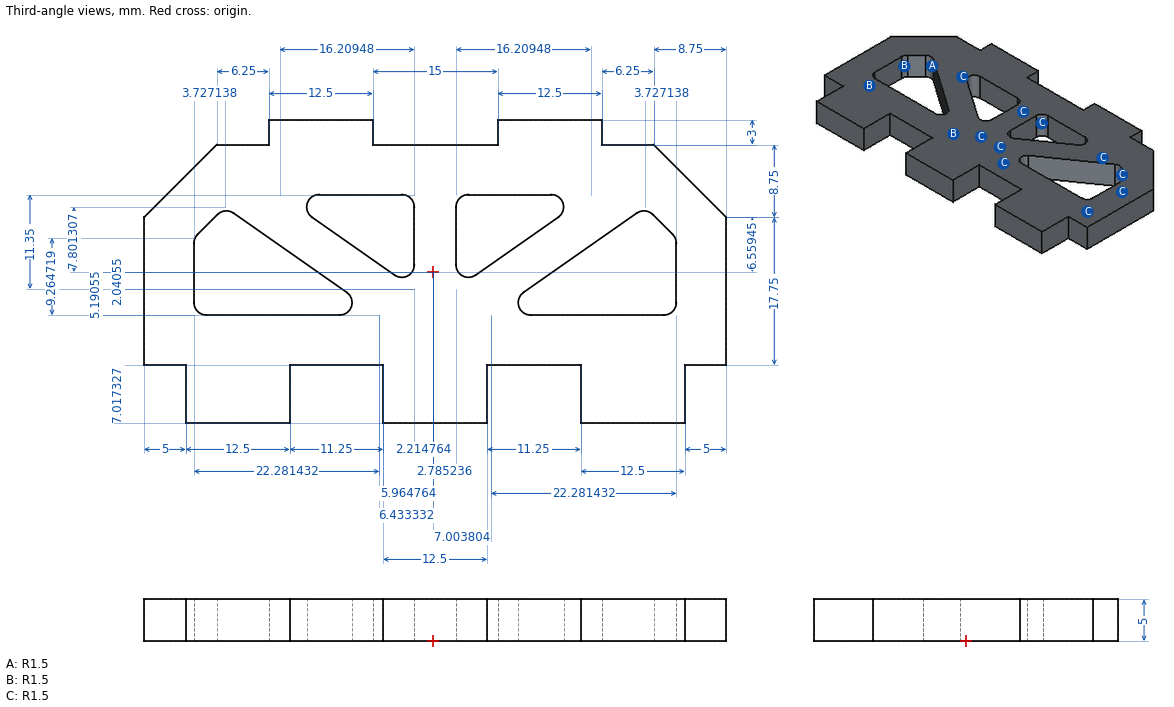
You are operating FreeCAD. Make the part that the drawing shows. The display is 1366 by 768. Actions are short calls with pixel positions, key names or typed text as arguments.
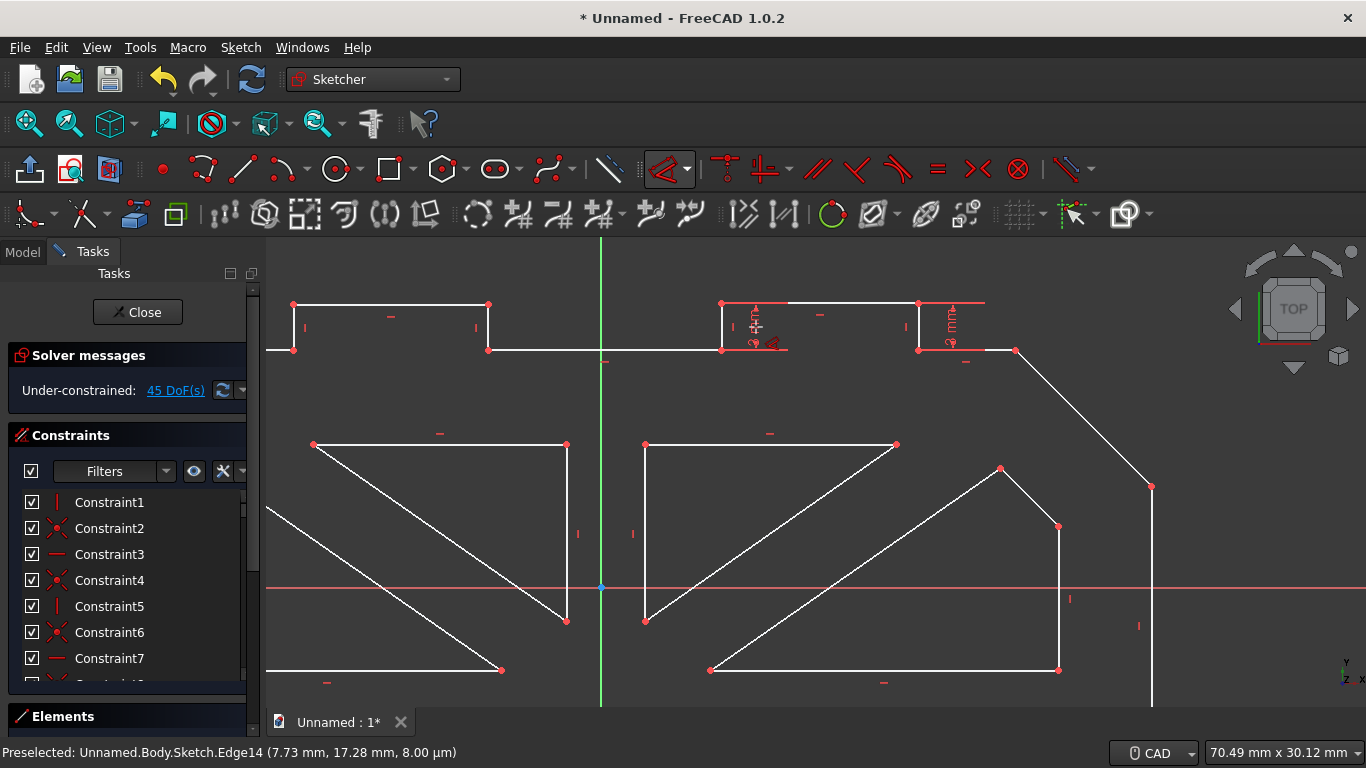
click(488, 336)
click(454, 327)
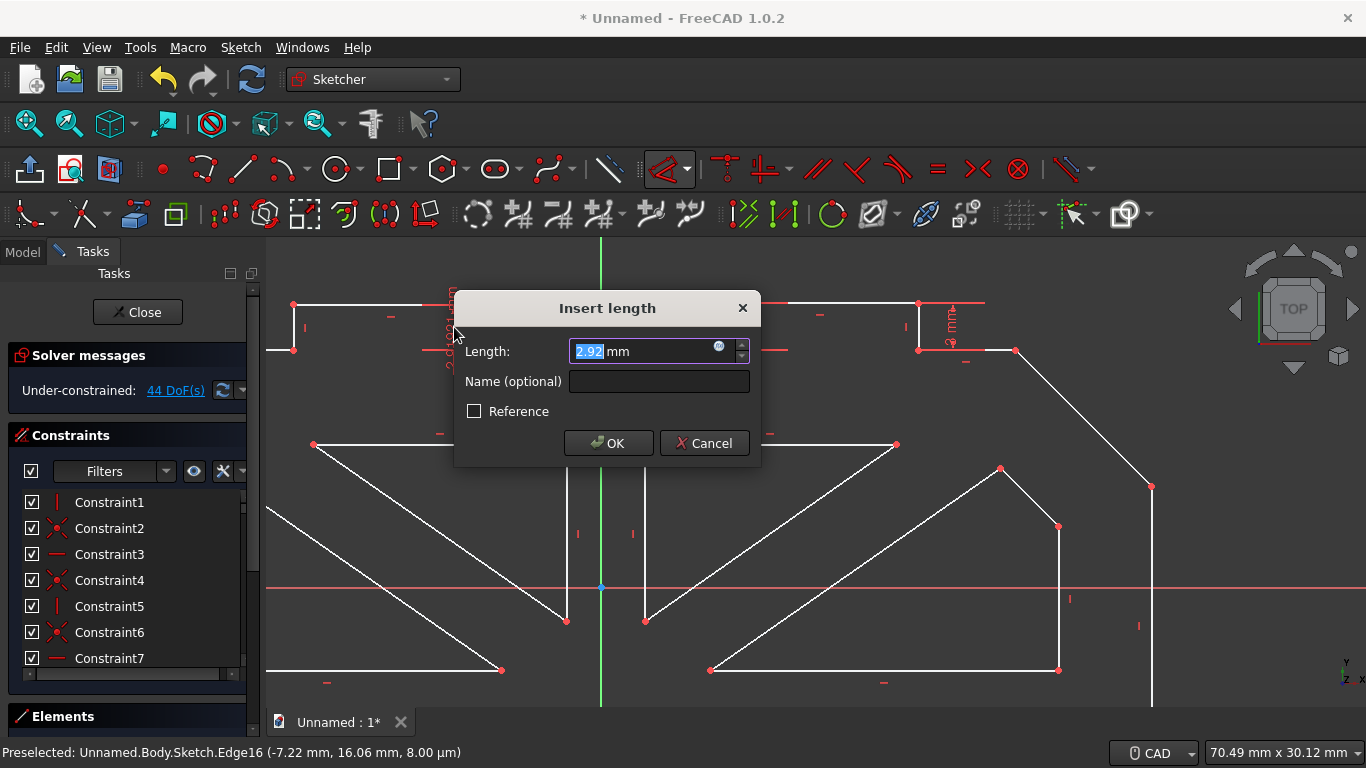
text(3)
key(Return)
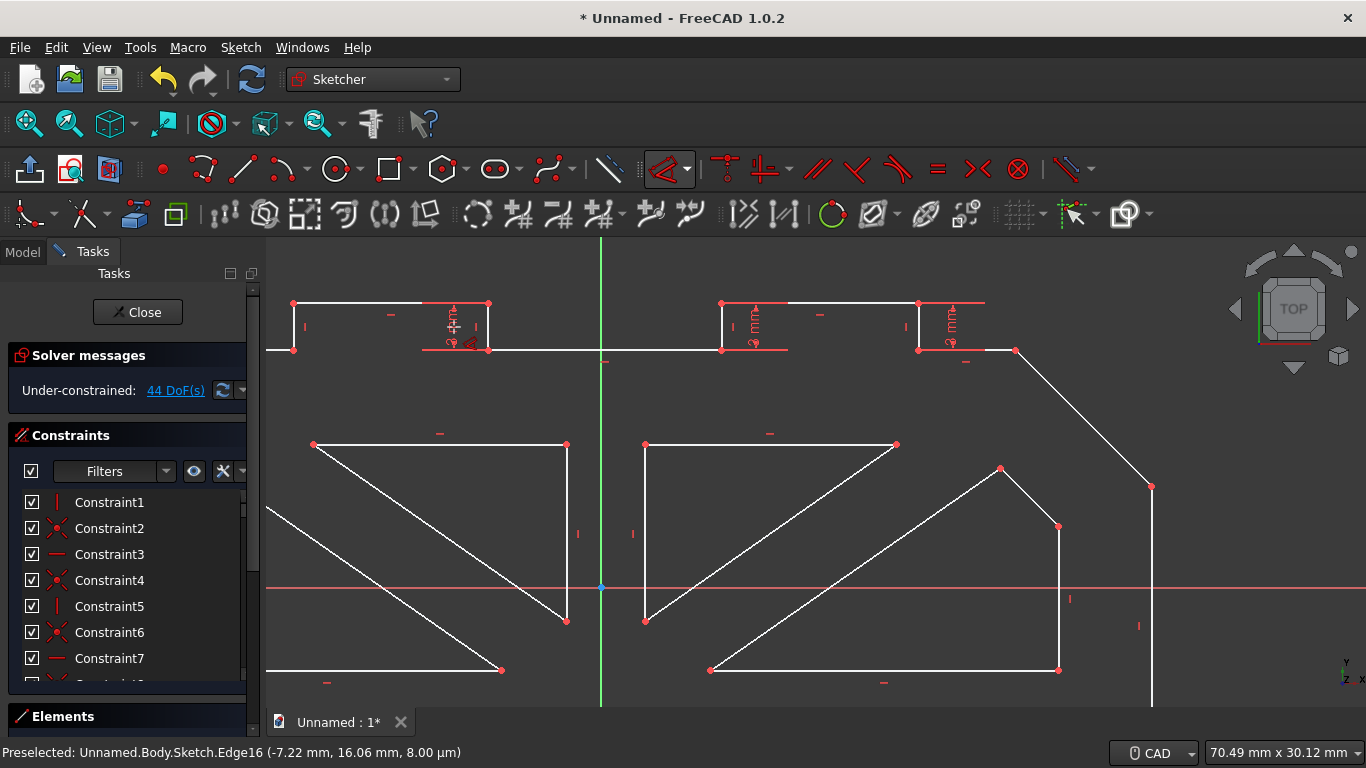
scroll(920, 332, down, 3)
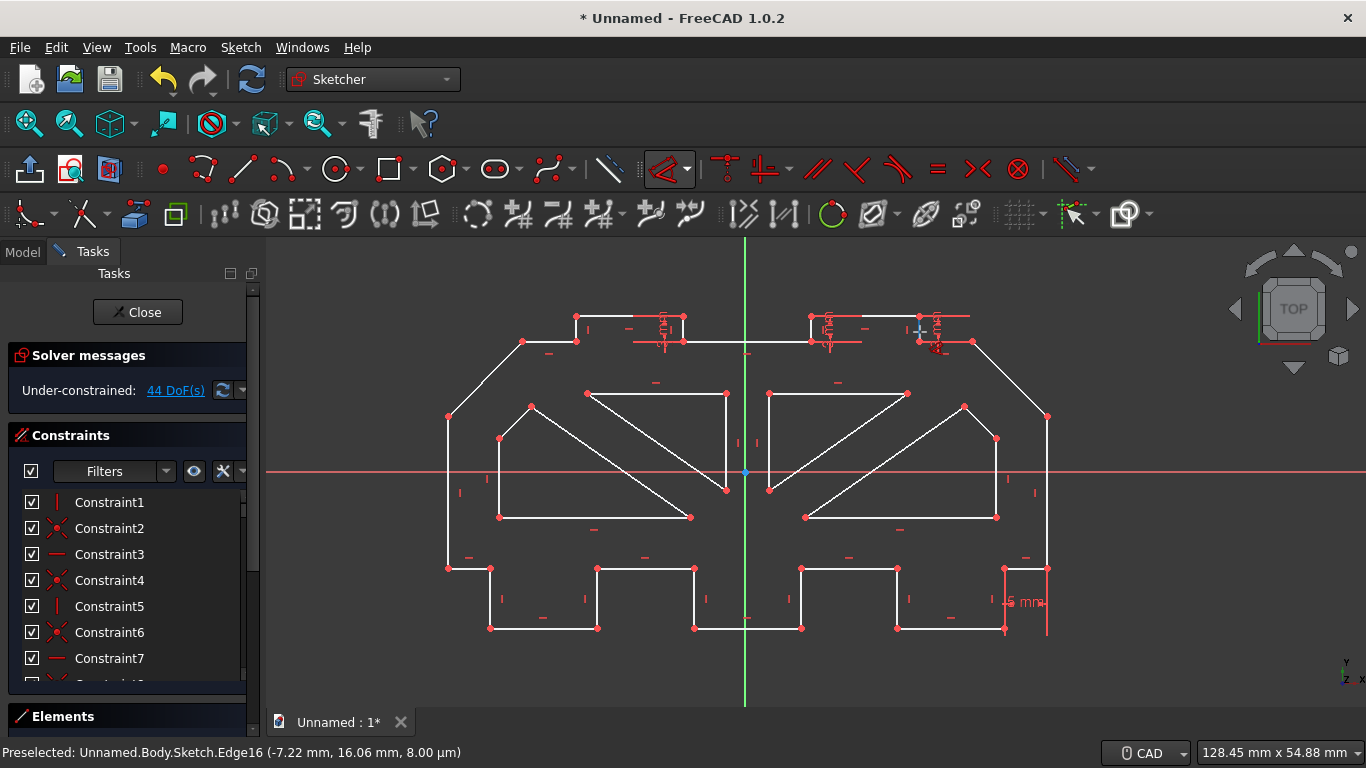
scroll(576, 324, up, 3)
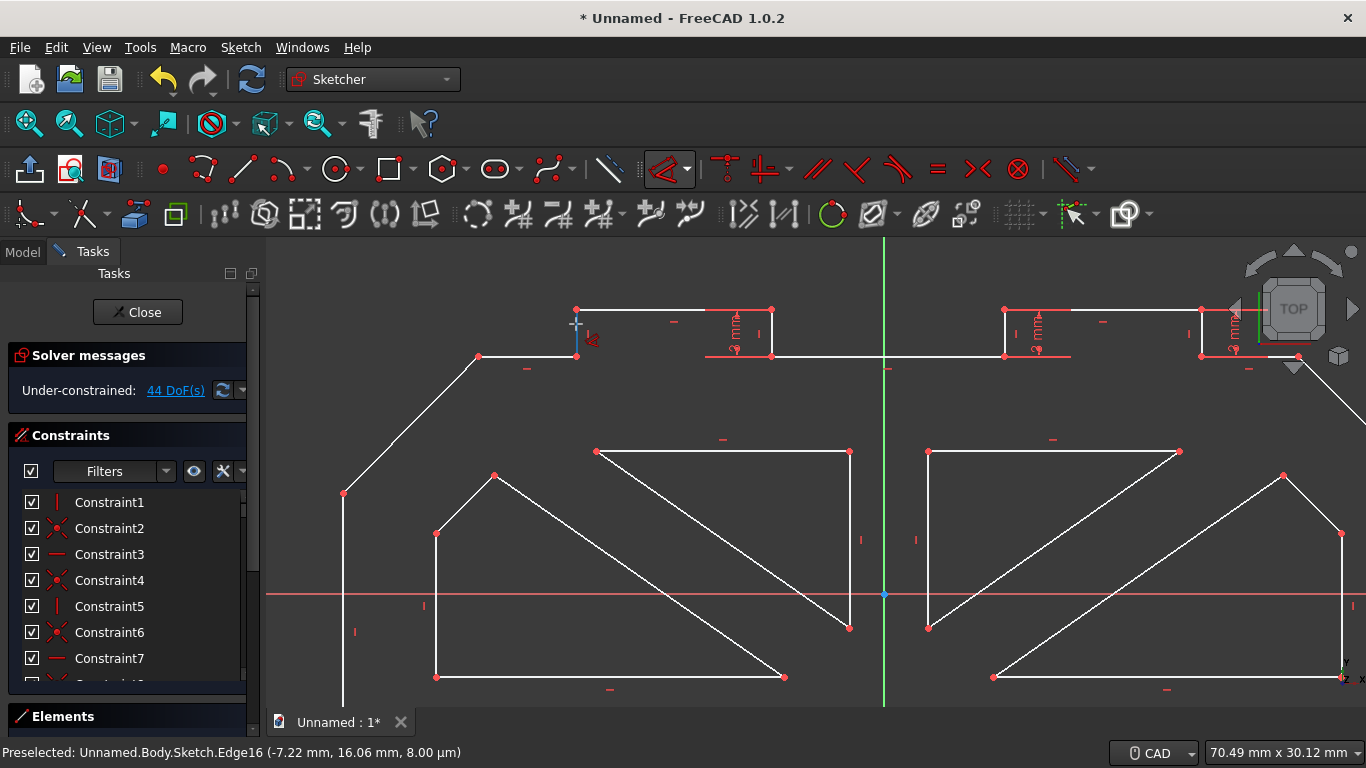
click(577, 324)
click(543, 333)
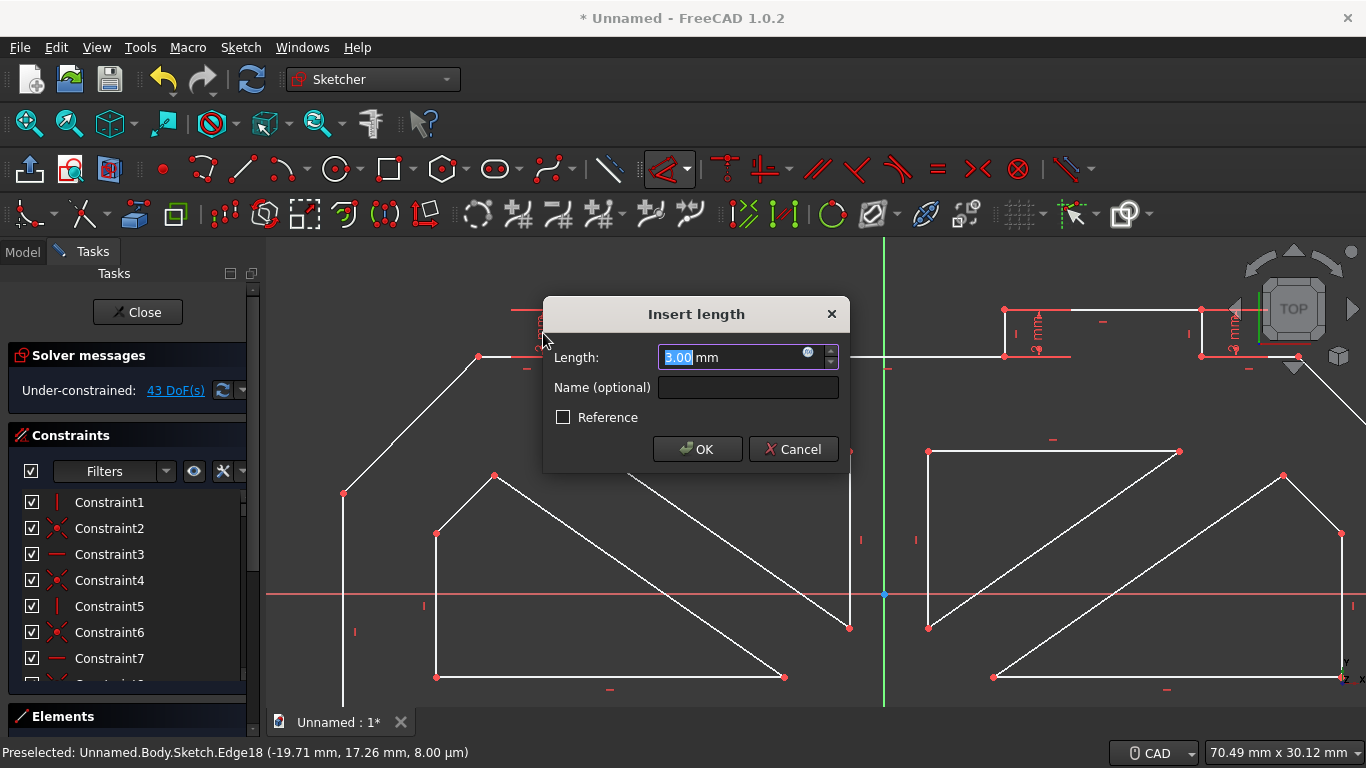
text(3)
key(Return)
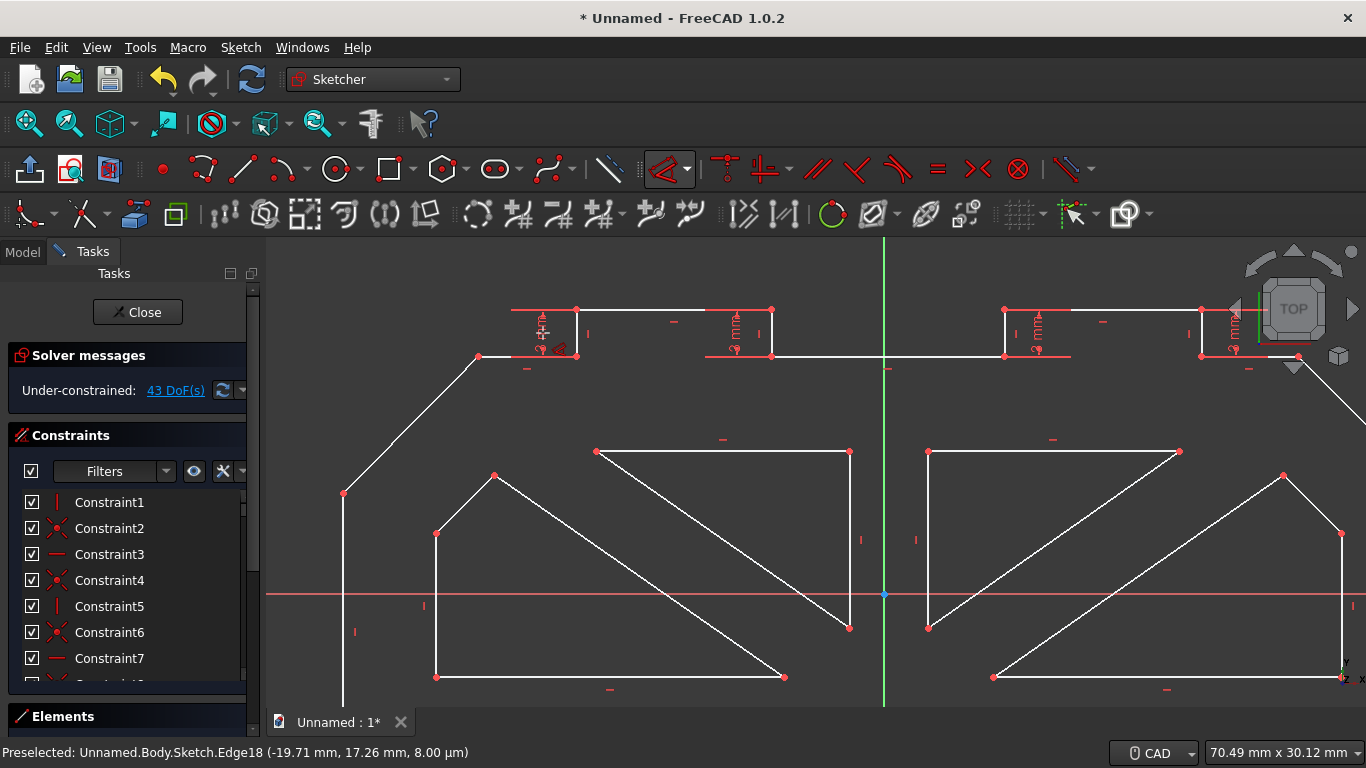
scroll(576, 324, down, 3)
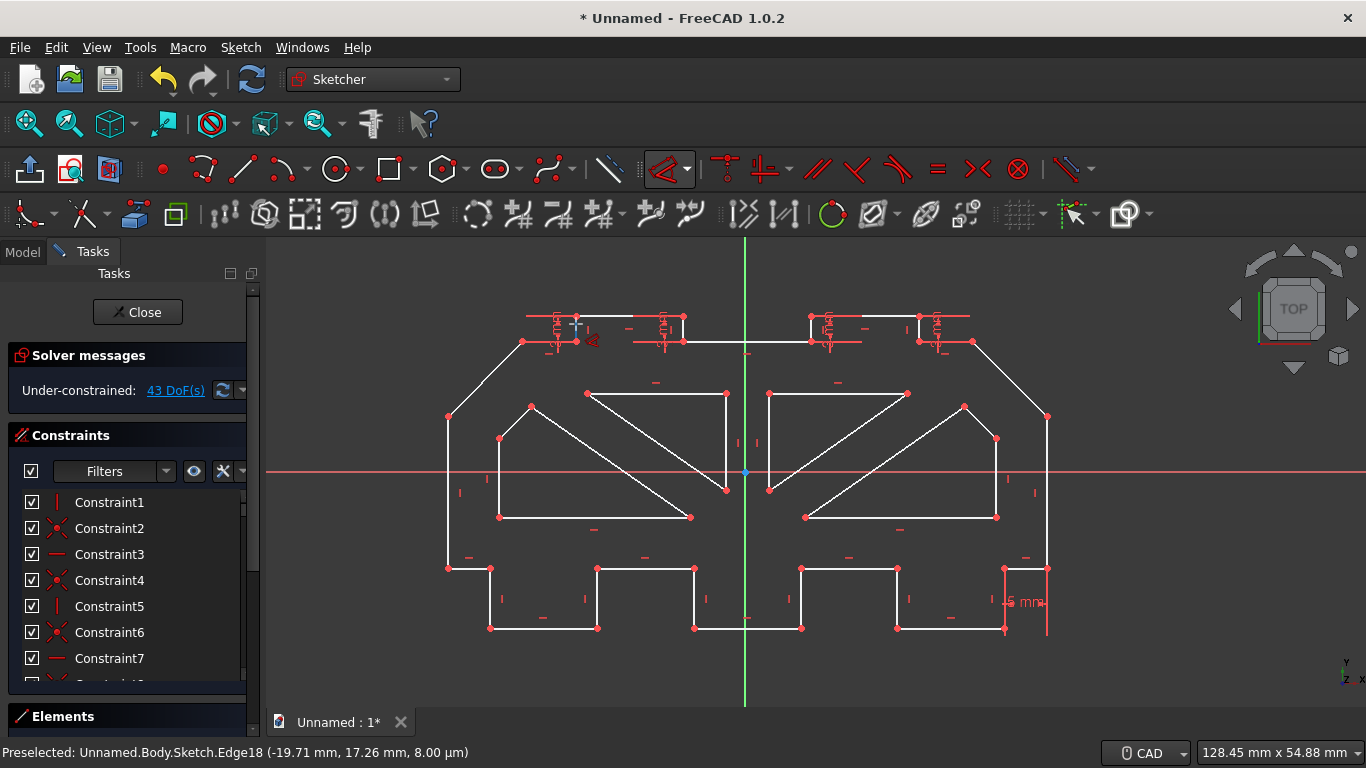
click(461, 569)
click(469, 603)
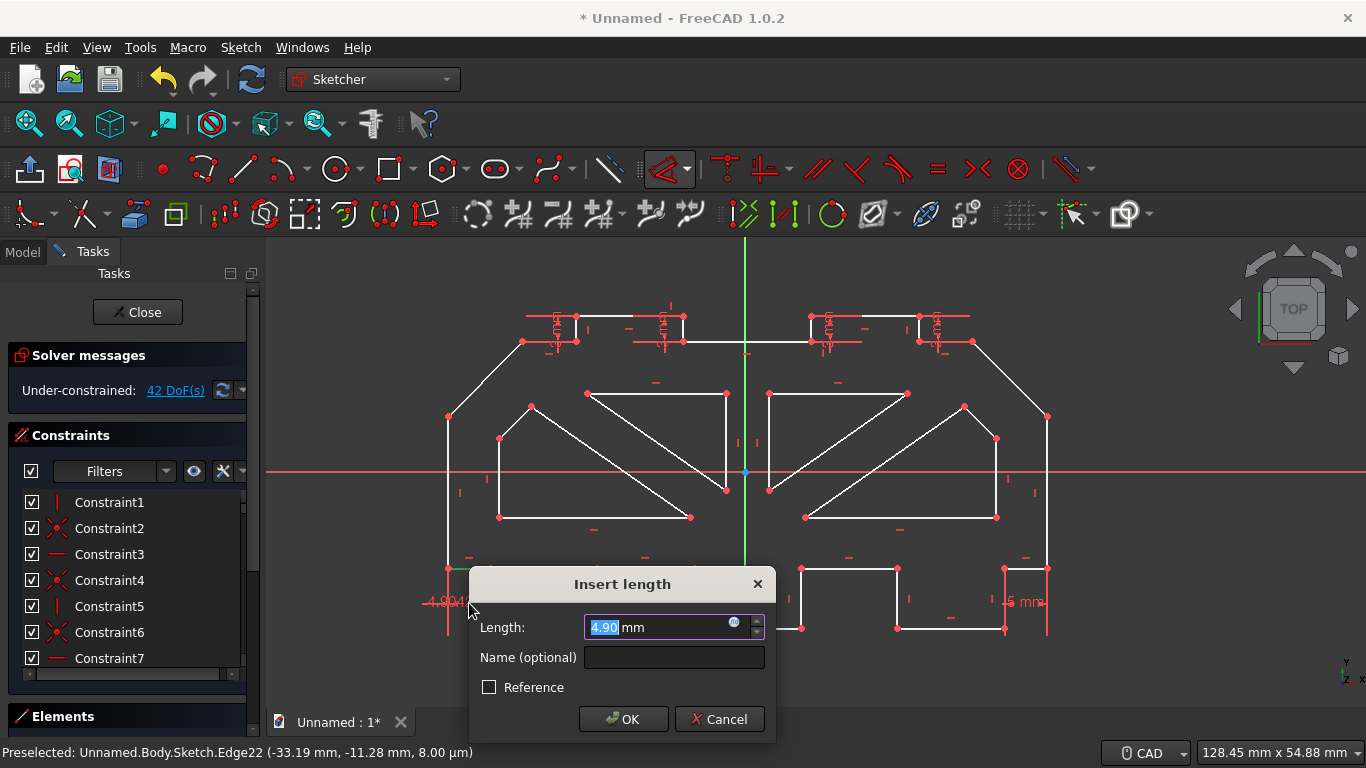
text(5)
key(Return)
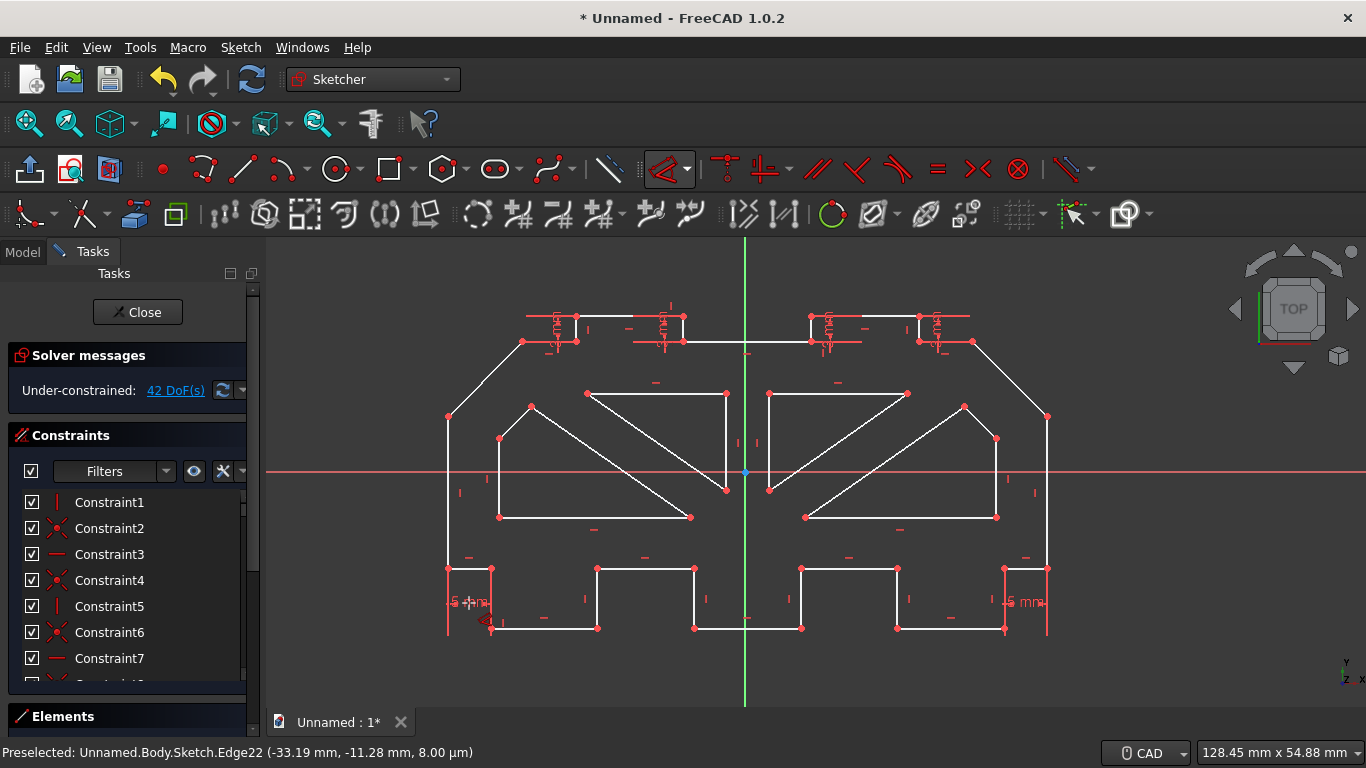
click(773, 342)
click(718, 308)